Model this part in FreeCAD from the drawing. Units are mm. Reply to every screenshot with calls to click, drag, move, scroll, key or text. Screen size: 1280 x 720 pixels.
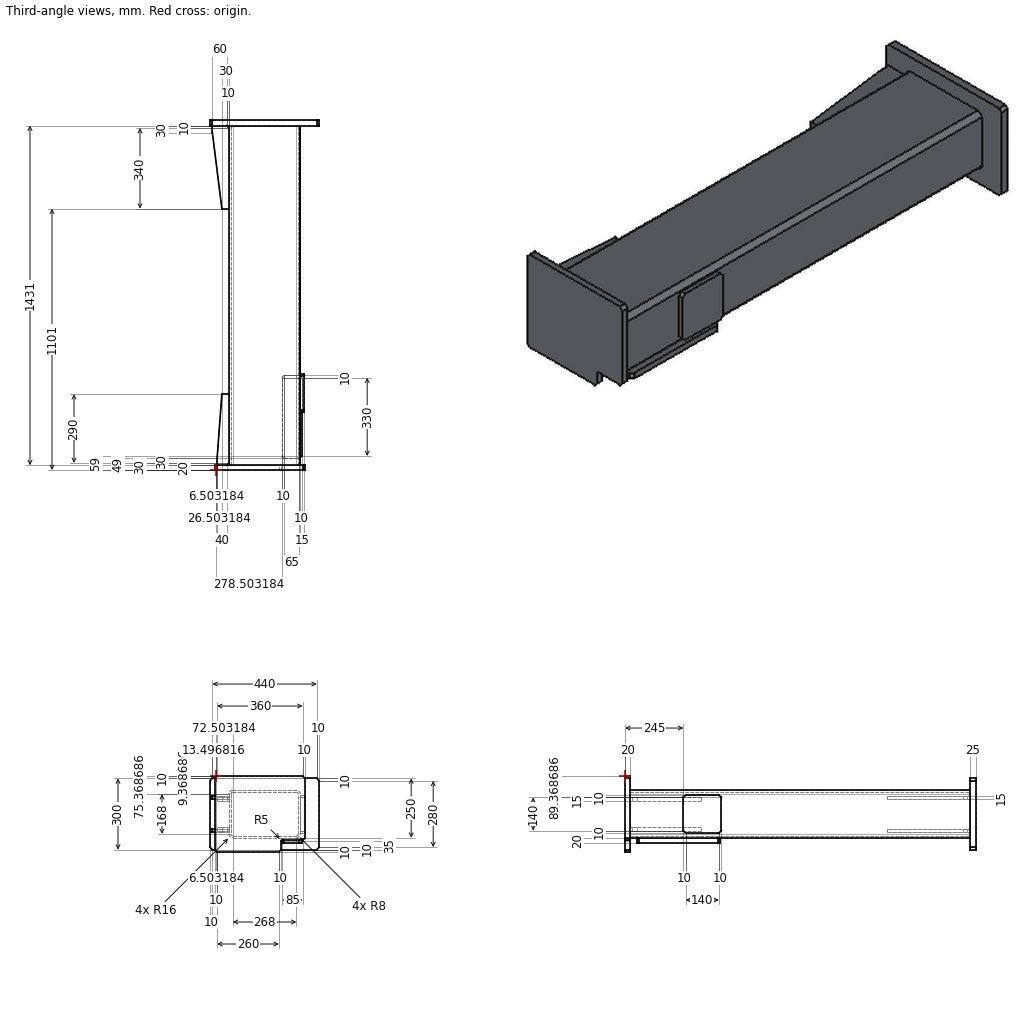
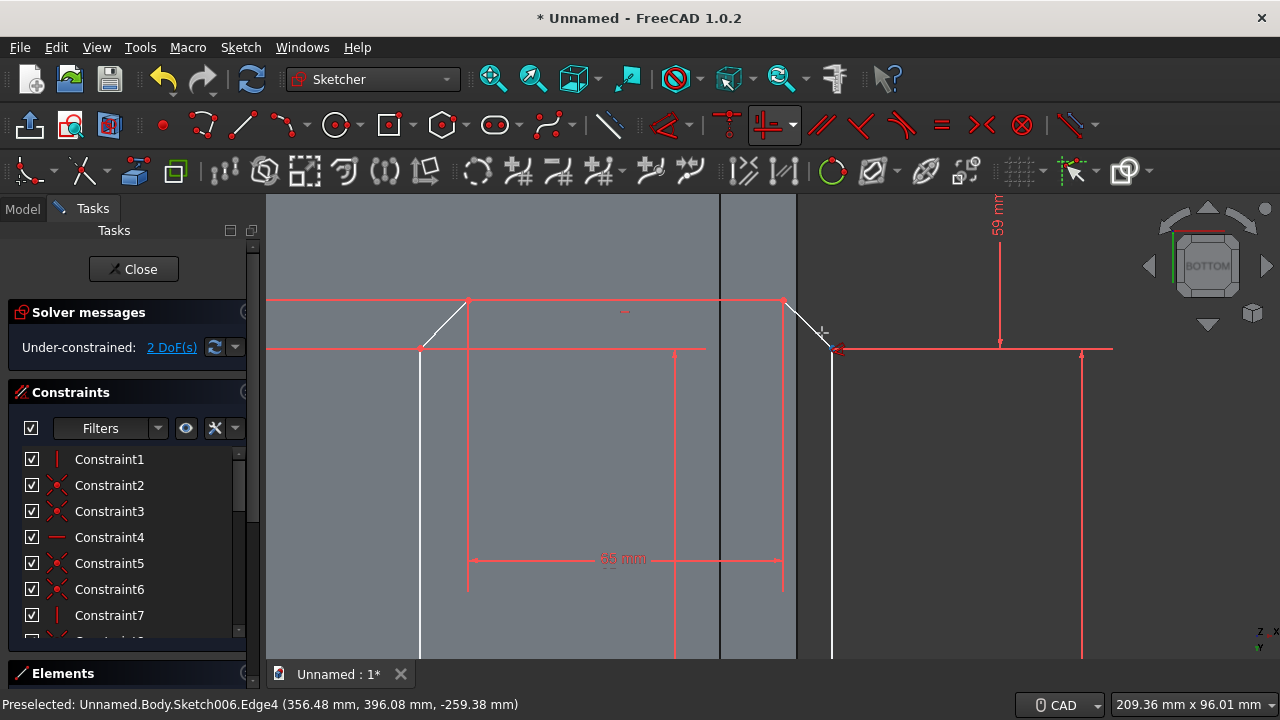
click(817, 334)
click(808, 266)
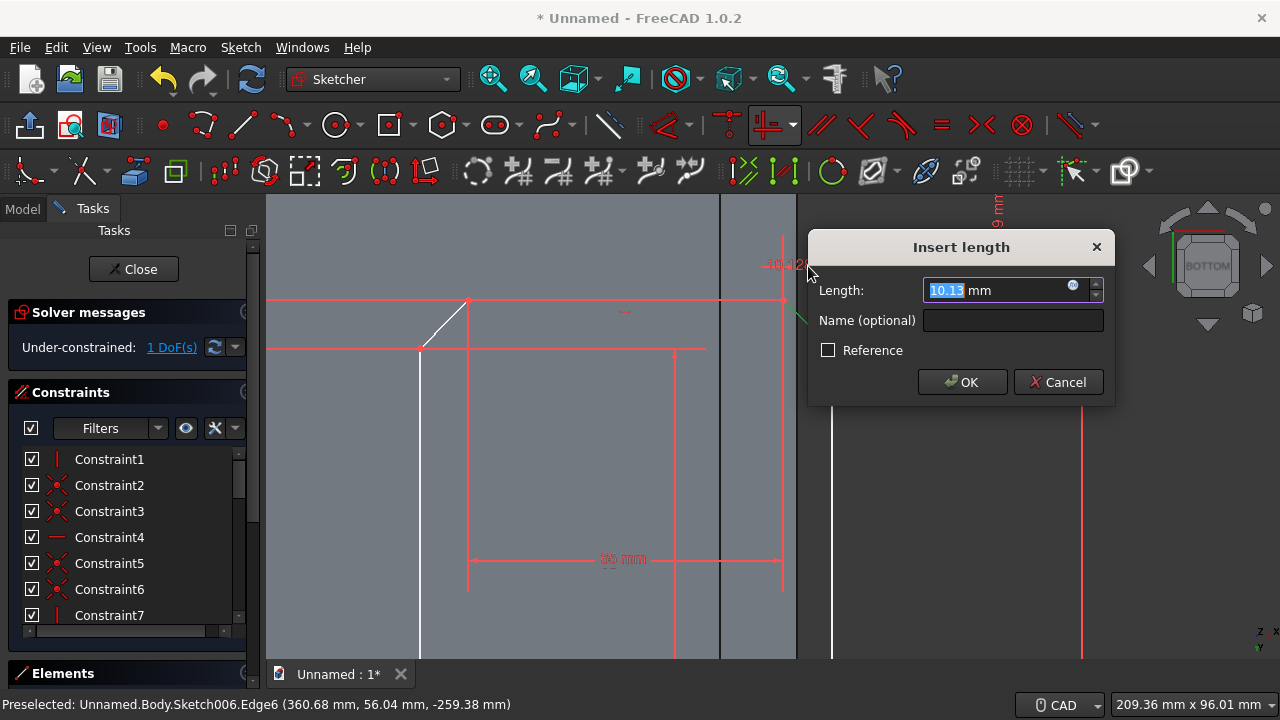
text(10)
key(Return)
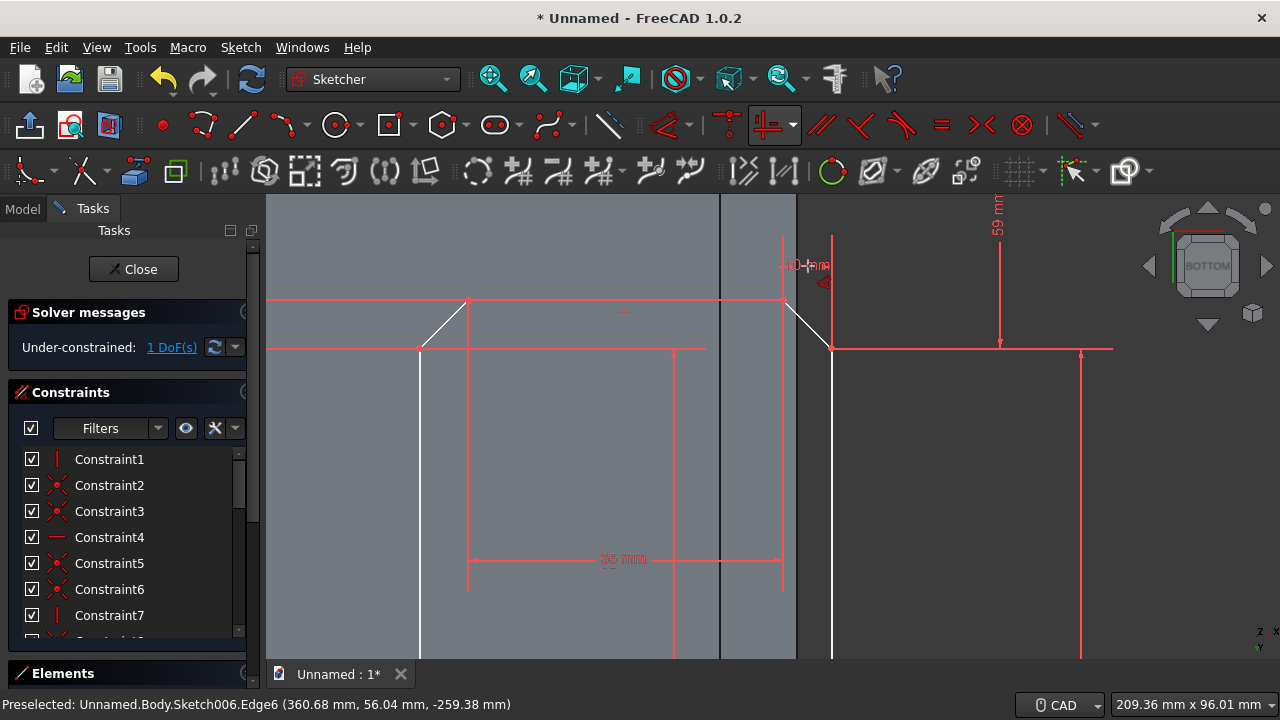
scroll(822, 332, down, 10)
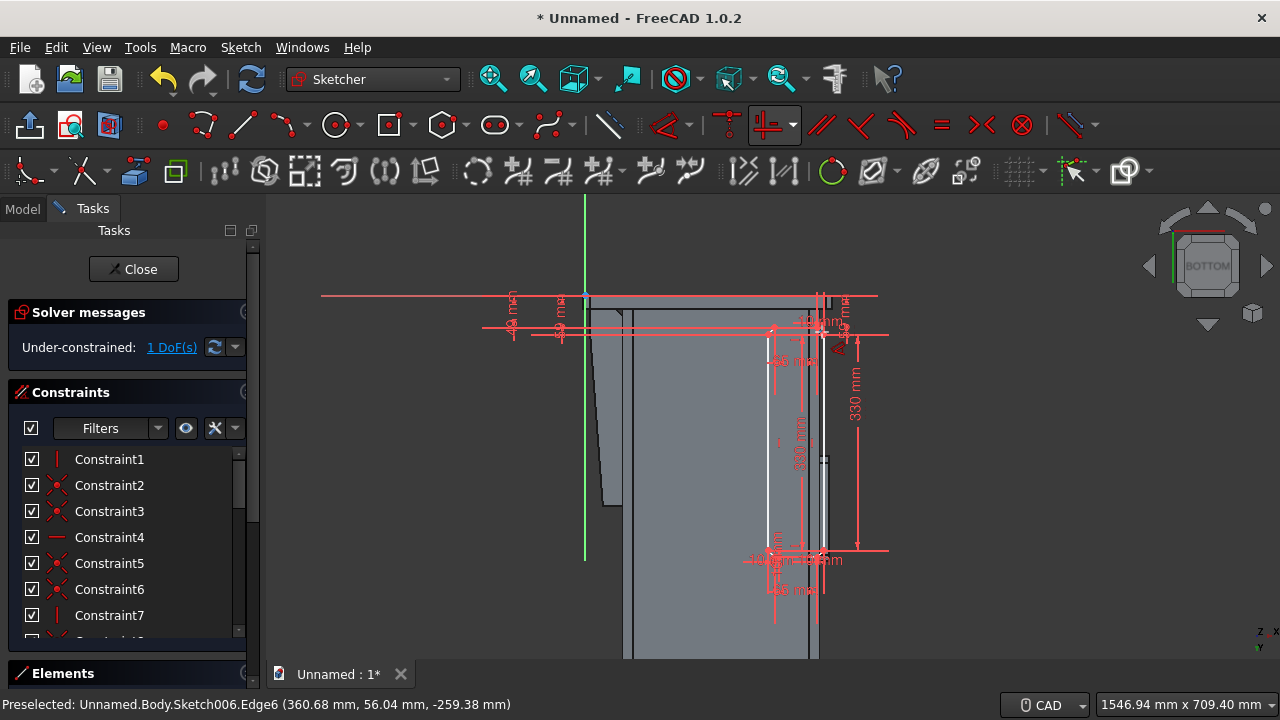
scroll(768, 335, up, 2)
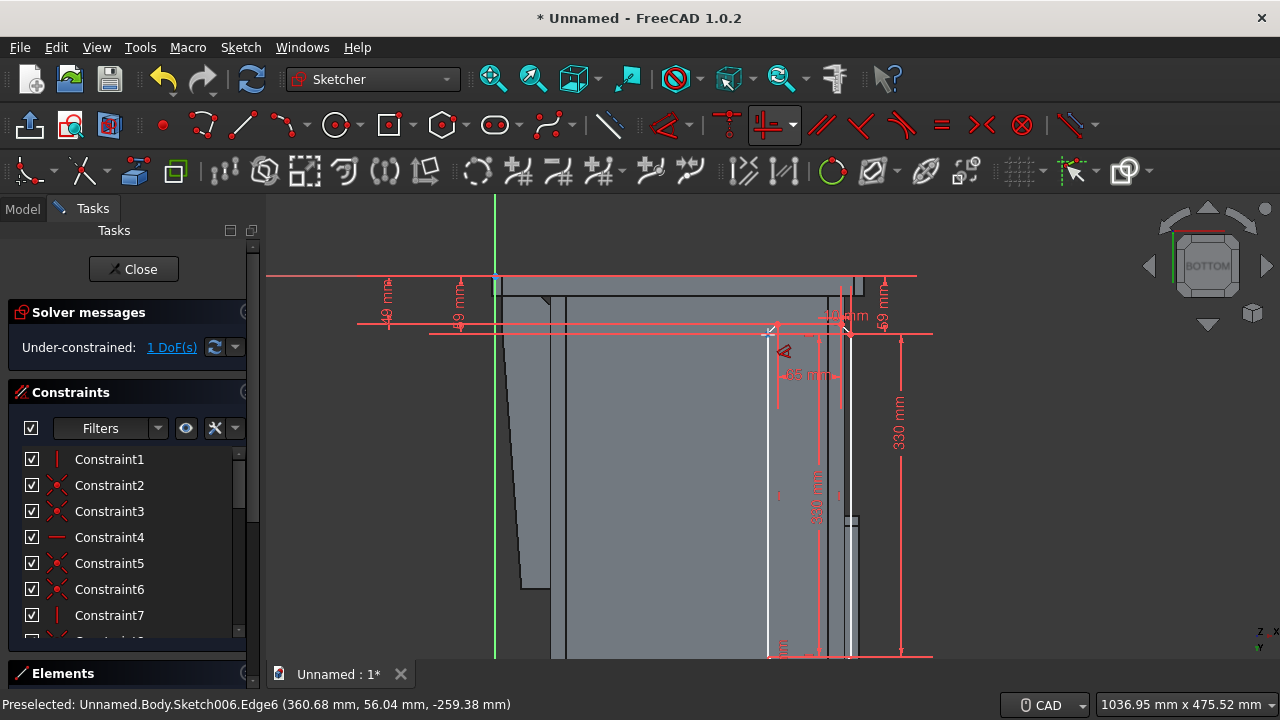
click(768, 334)
click(632, 242)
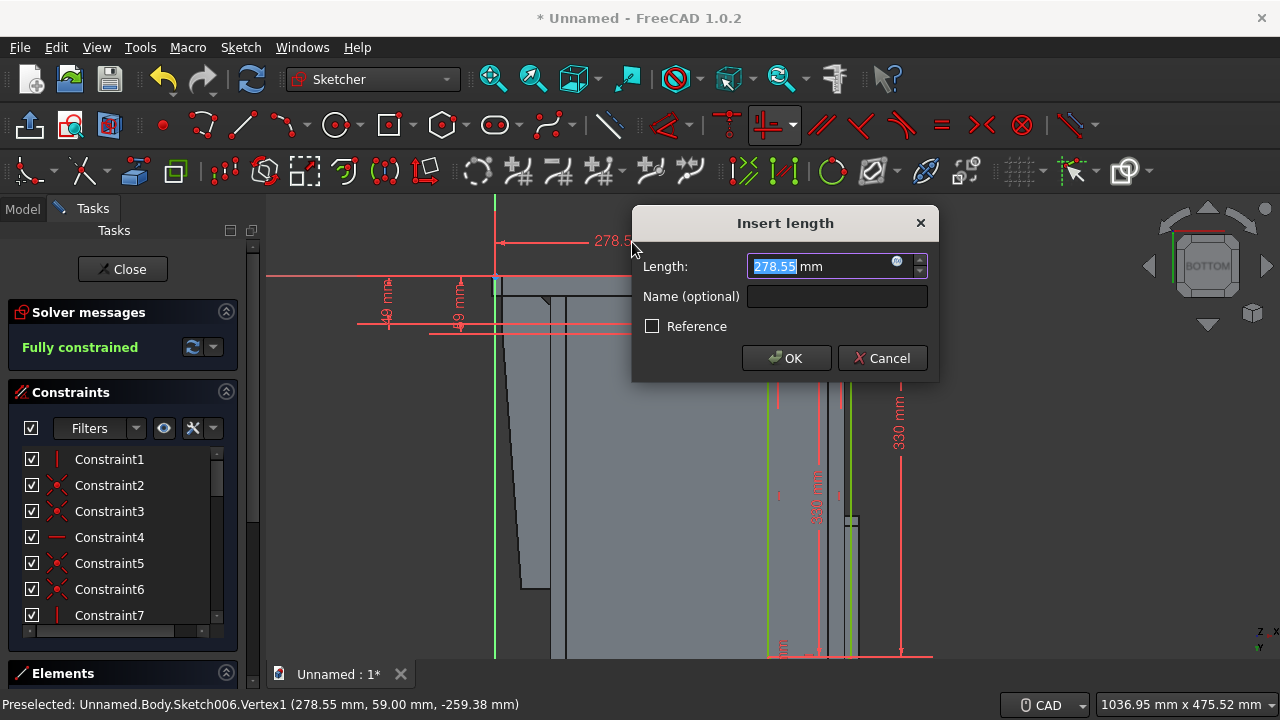
text(278.503184)
key(Return)
key(Escape)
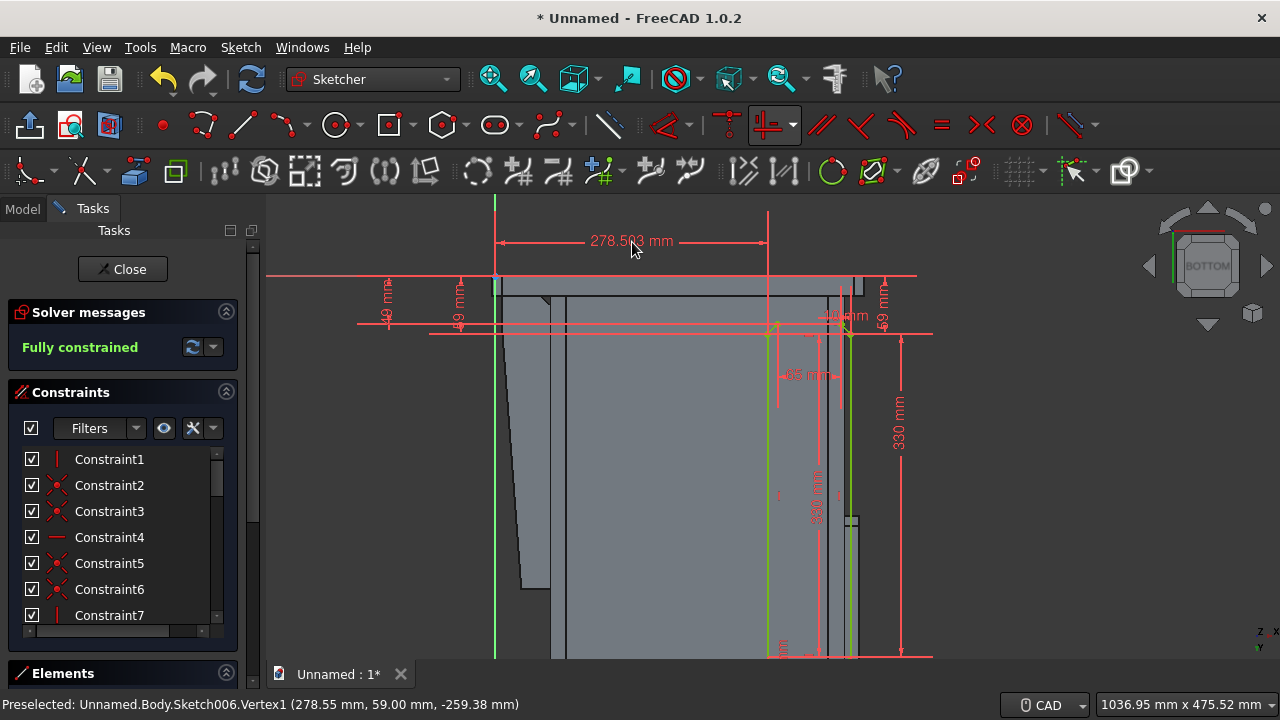
click(123, 269)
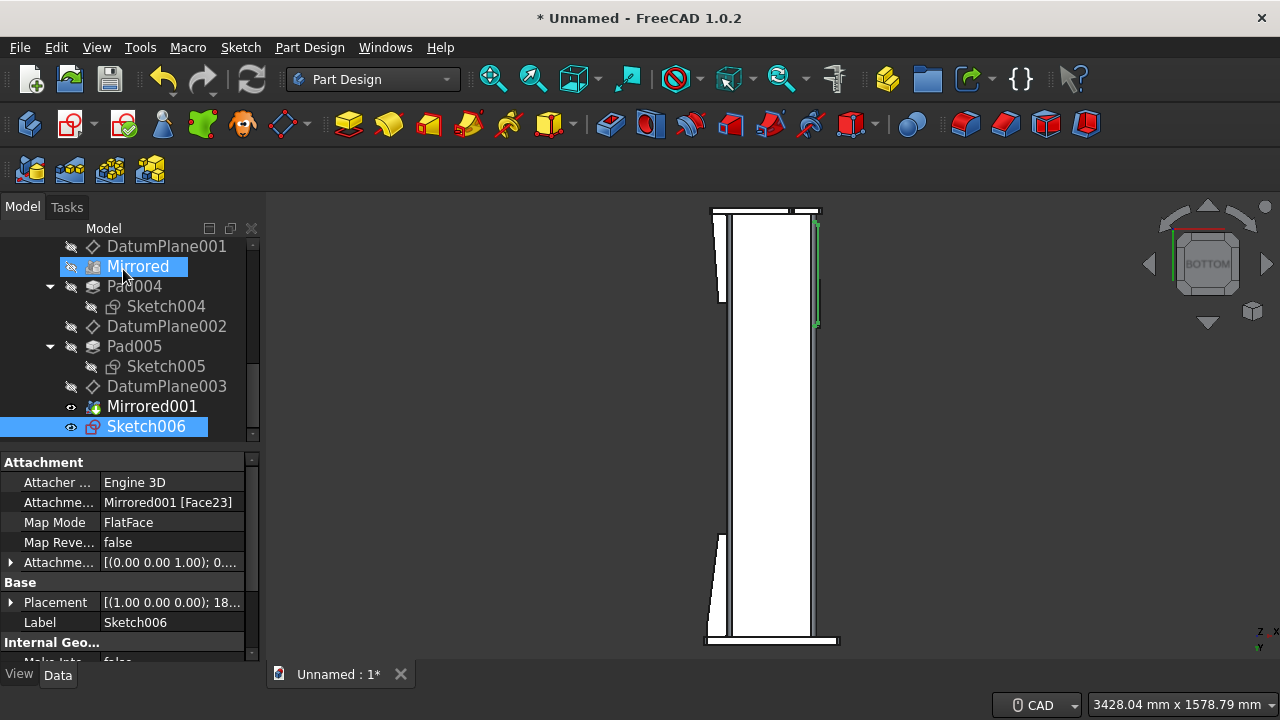
click(350, 124)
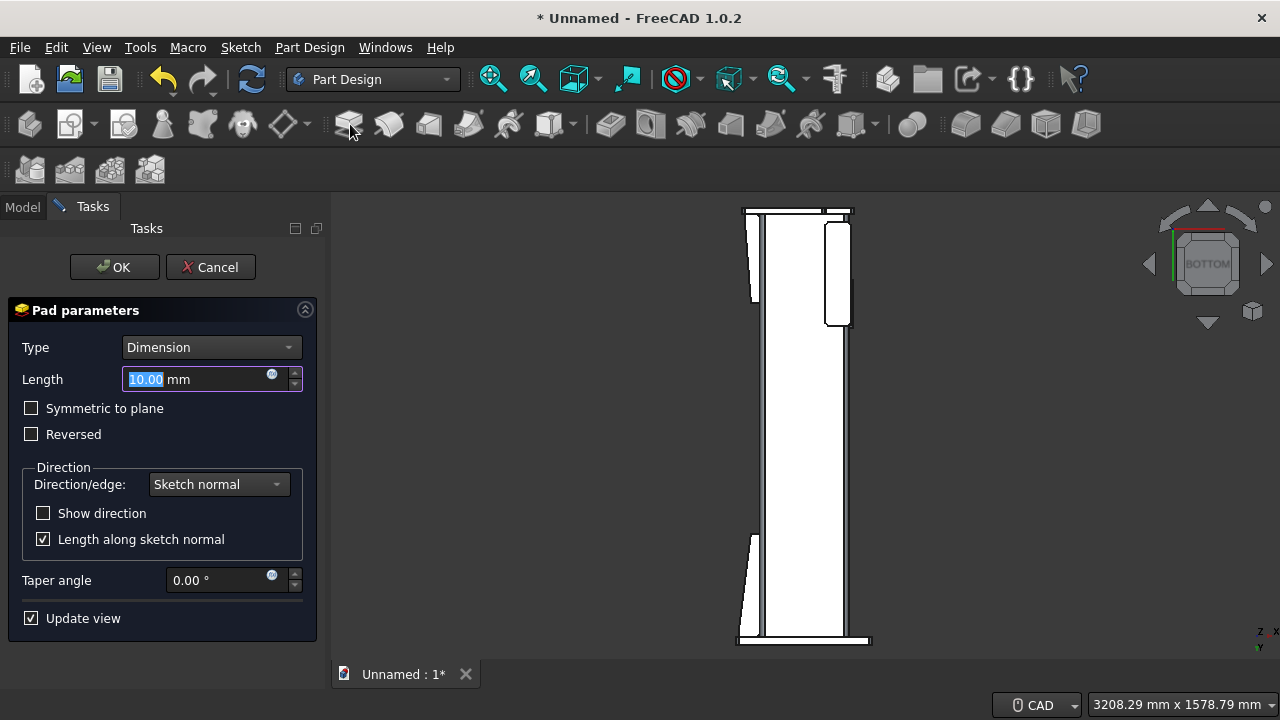
text(20)
key(Tab)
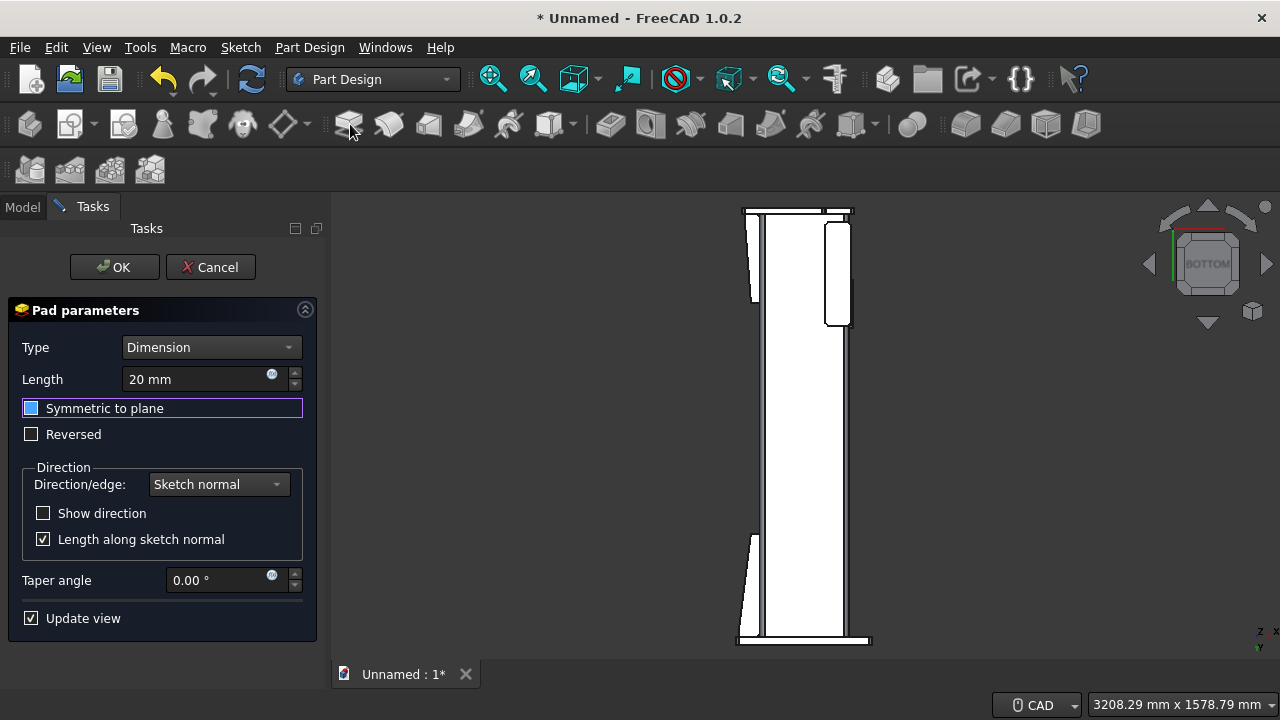
click(115, 267)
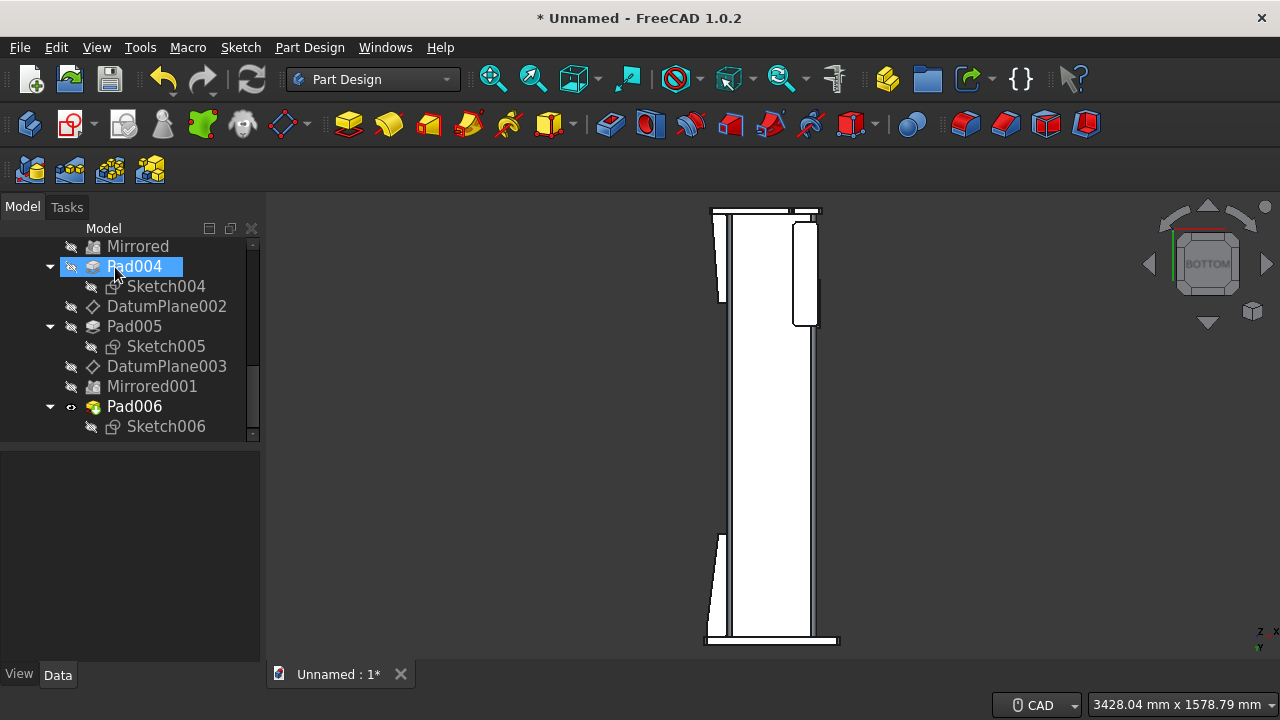
key(0)